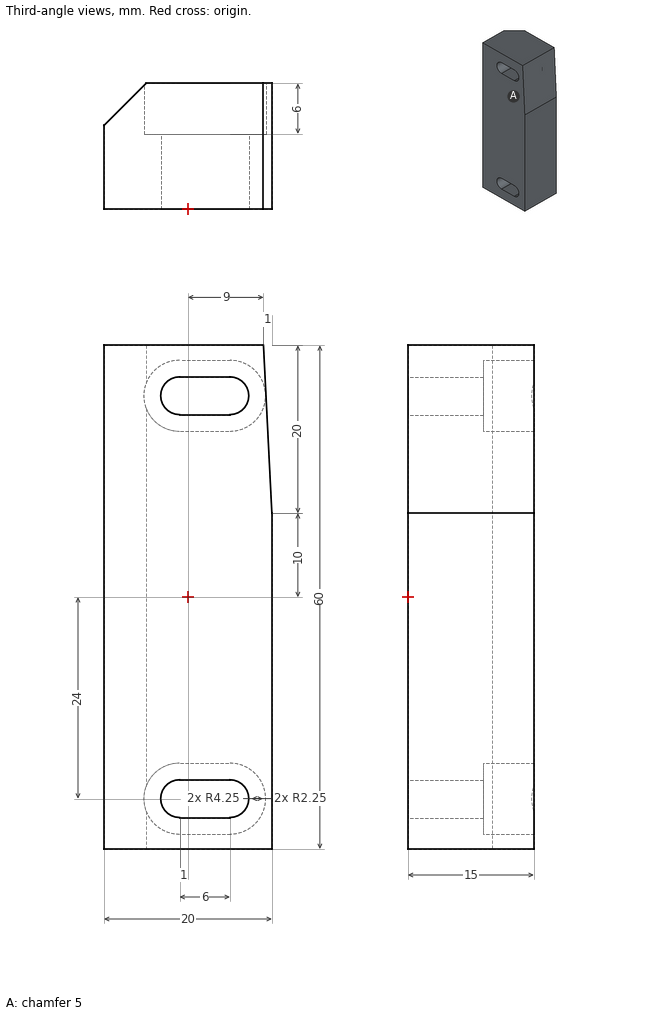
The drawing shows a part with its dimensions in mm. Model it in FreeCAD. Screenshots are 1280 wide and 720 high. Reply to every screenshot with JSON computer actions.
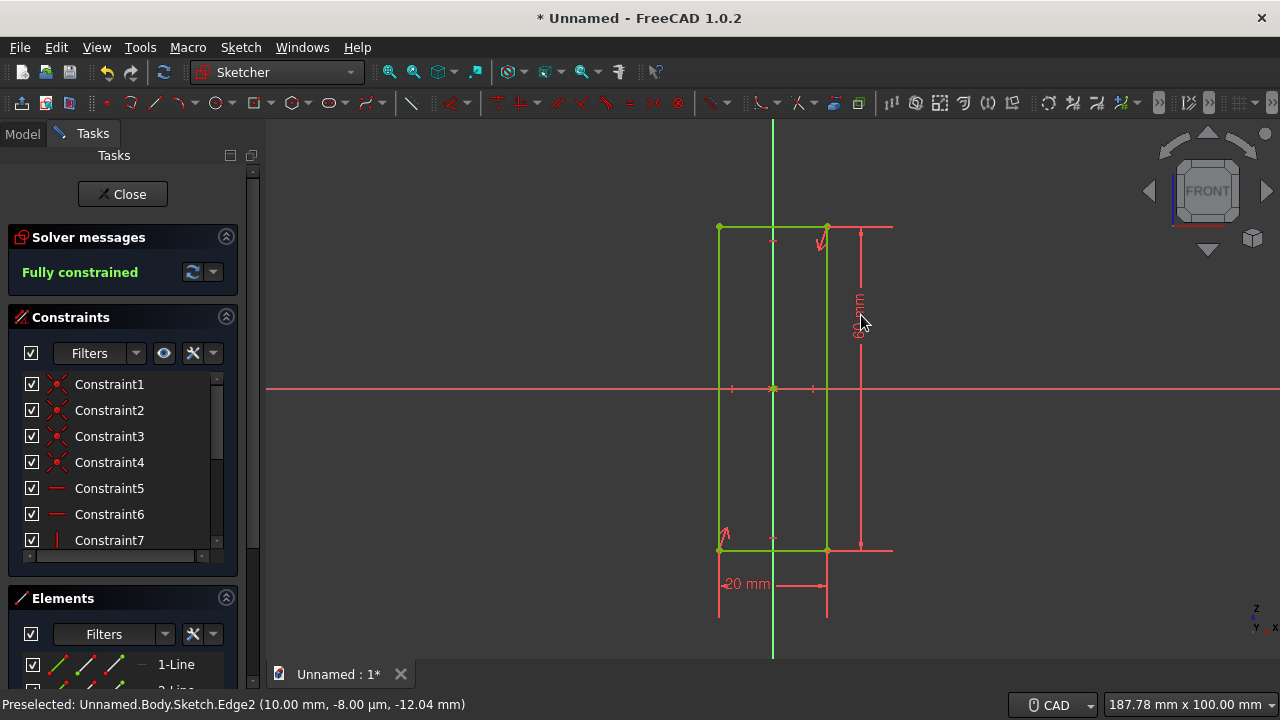
{"action": "left_click", "coordinate": [123, 194]}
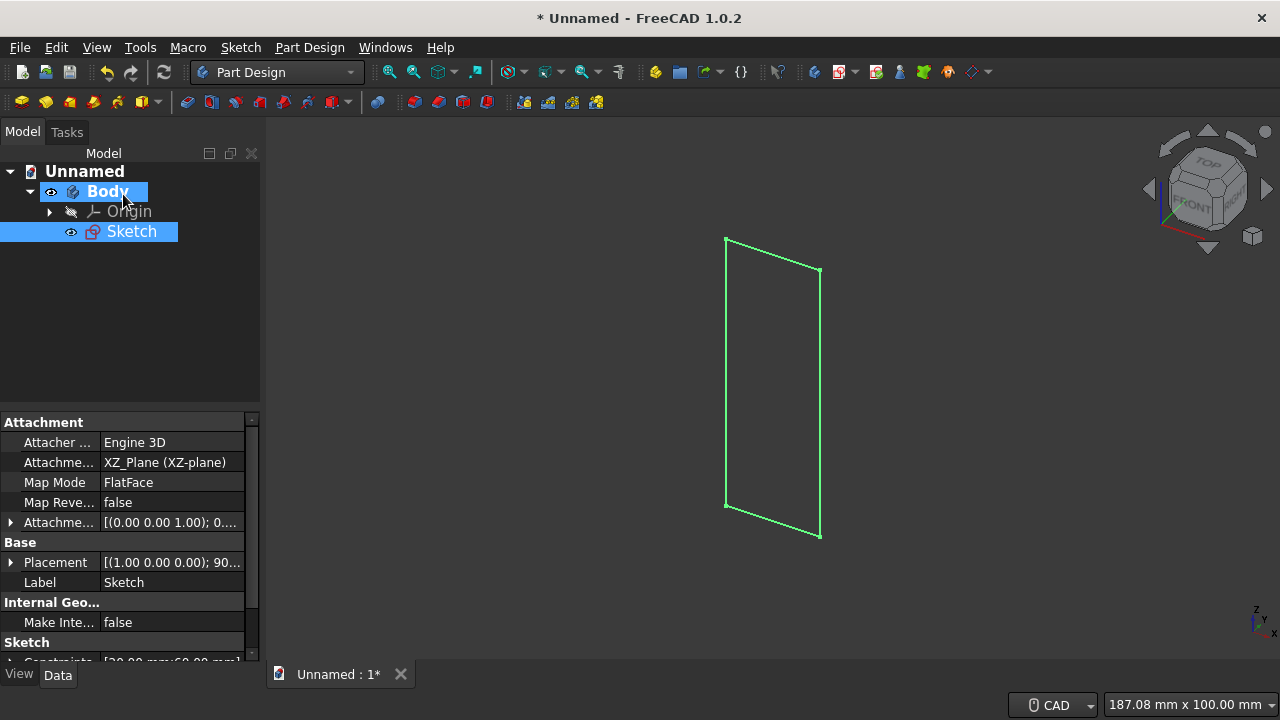
{"action": "left_click", "coordinate": [22, 102]}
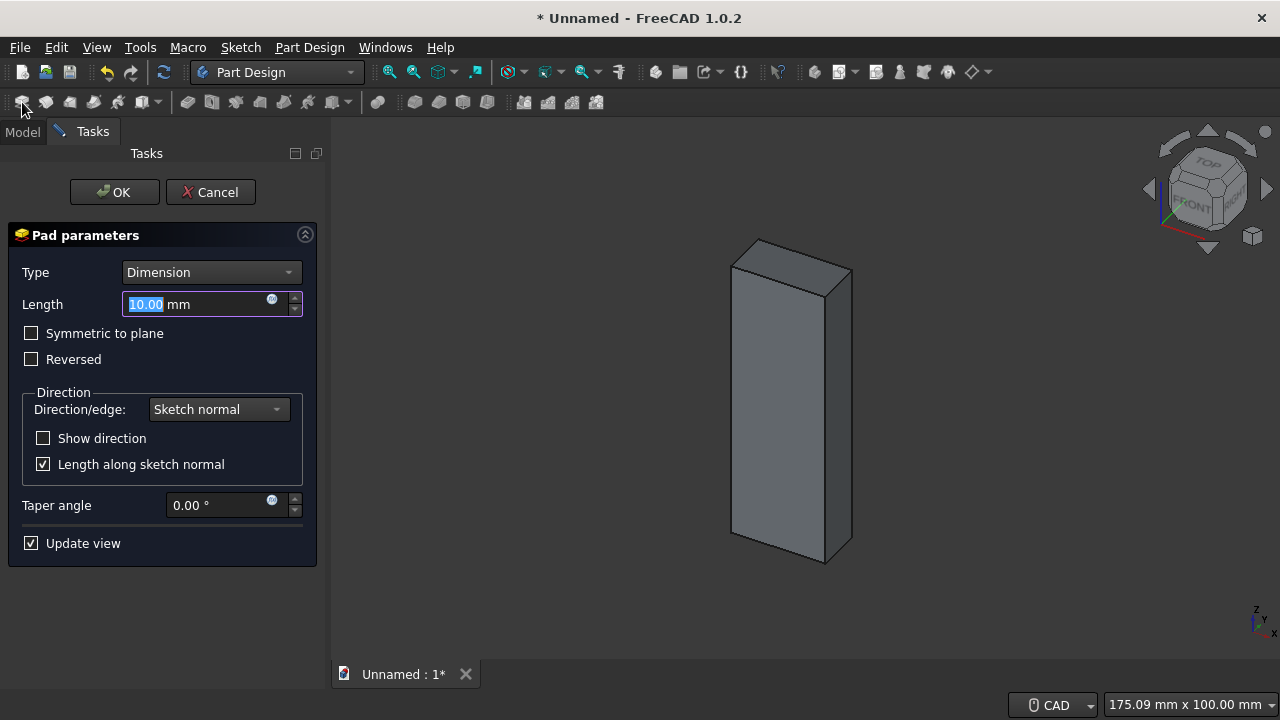
{"action": "type", "text": "15"}
{"action": "key", "text": "Tab"}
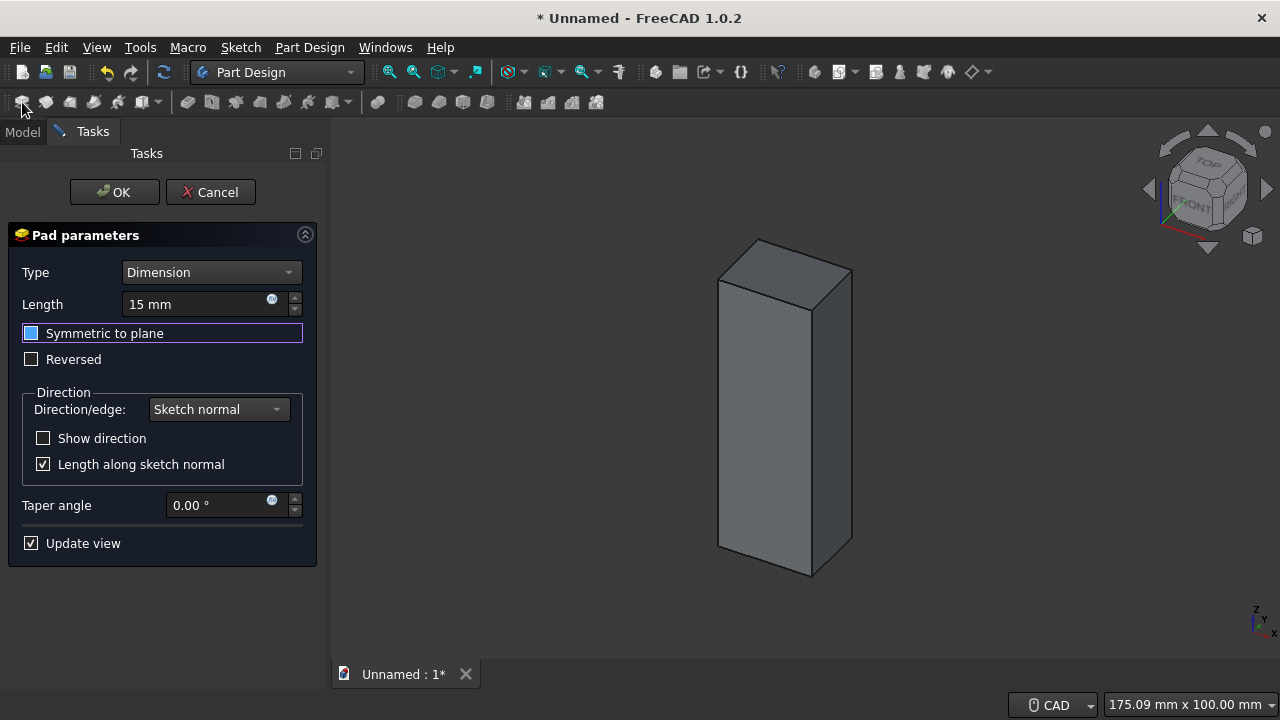
{"action": "left_click", "coordinate": [30, 359]}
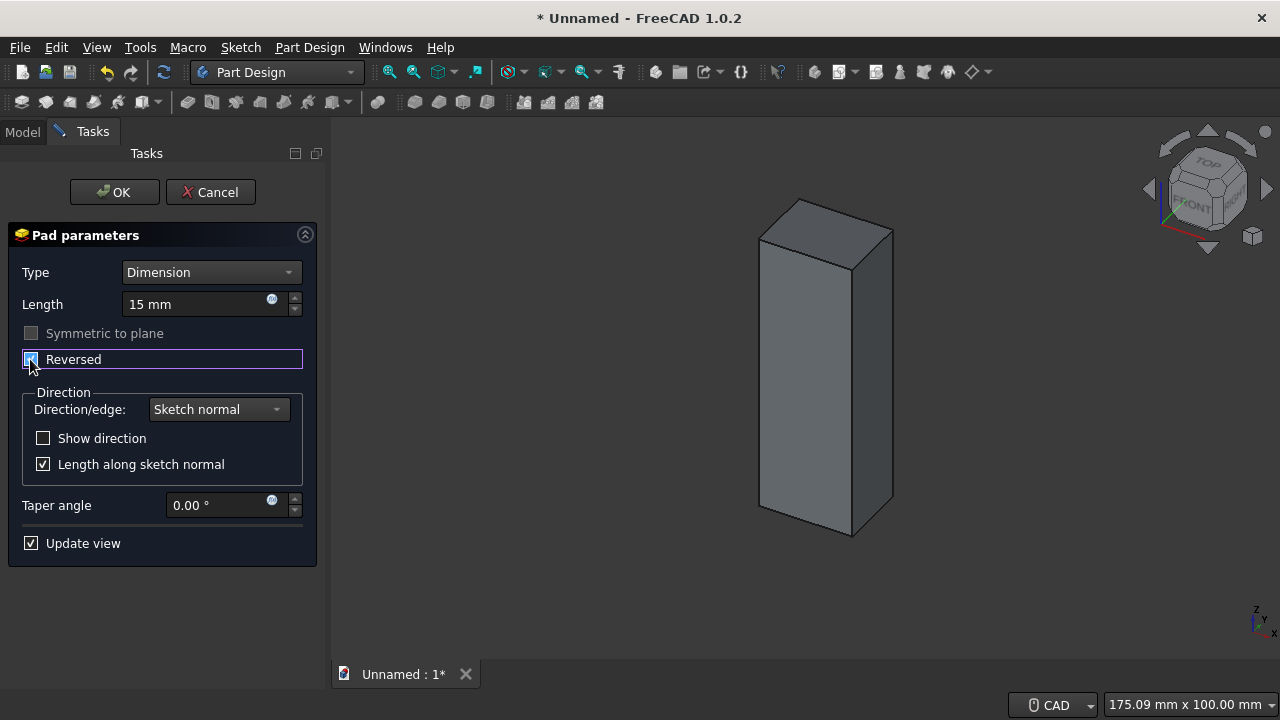
{"action": "left_click", "coordinate": [115, 192]}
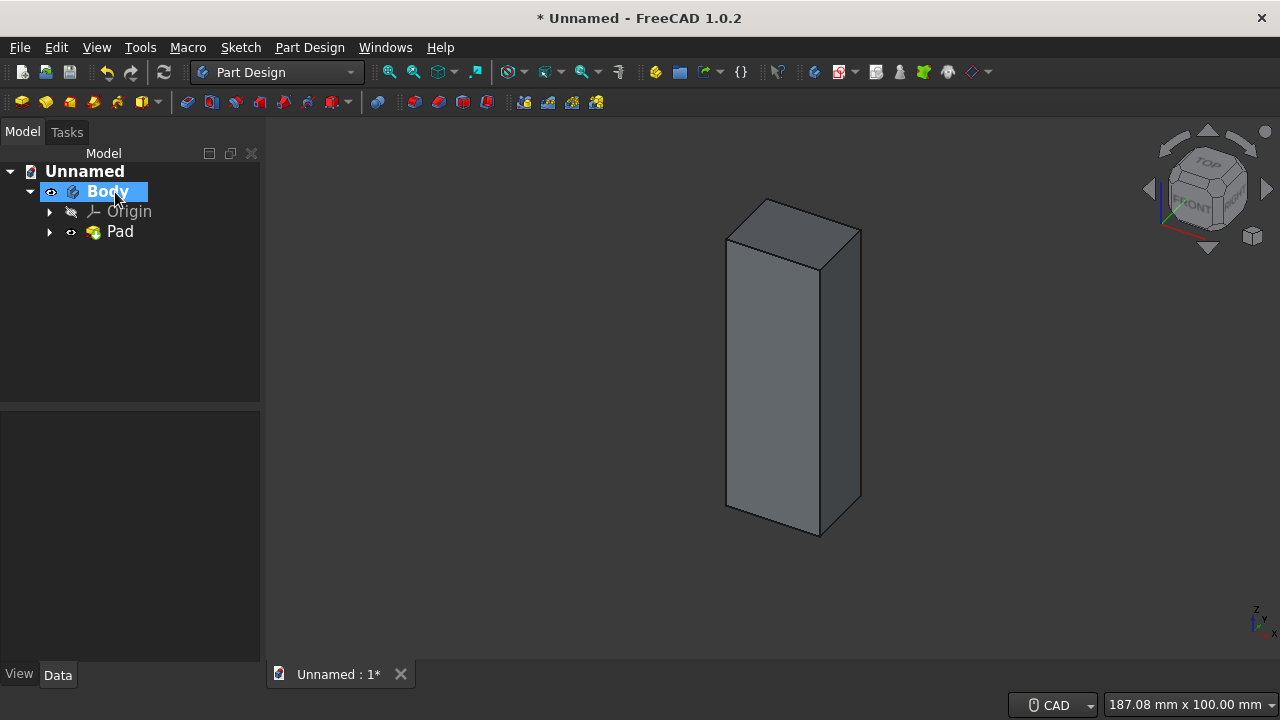
{"action": "key", "text": "0"}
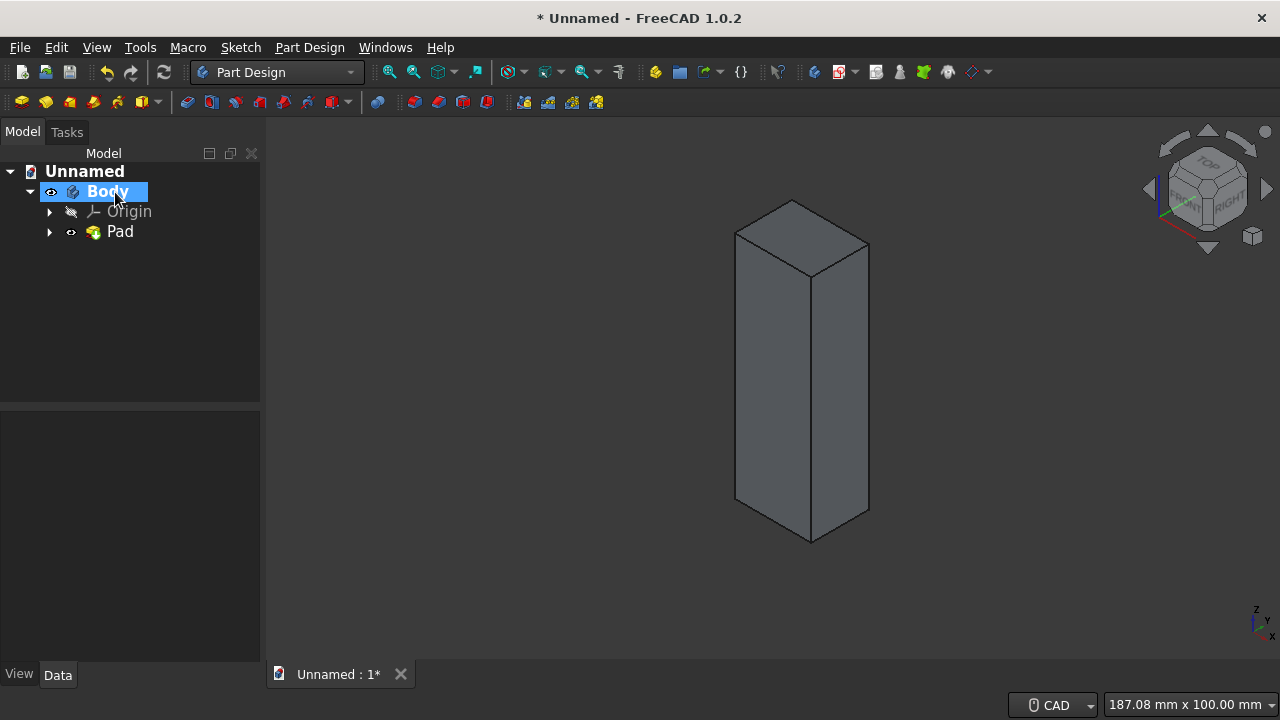
{"action": "key", "text": "2"}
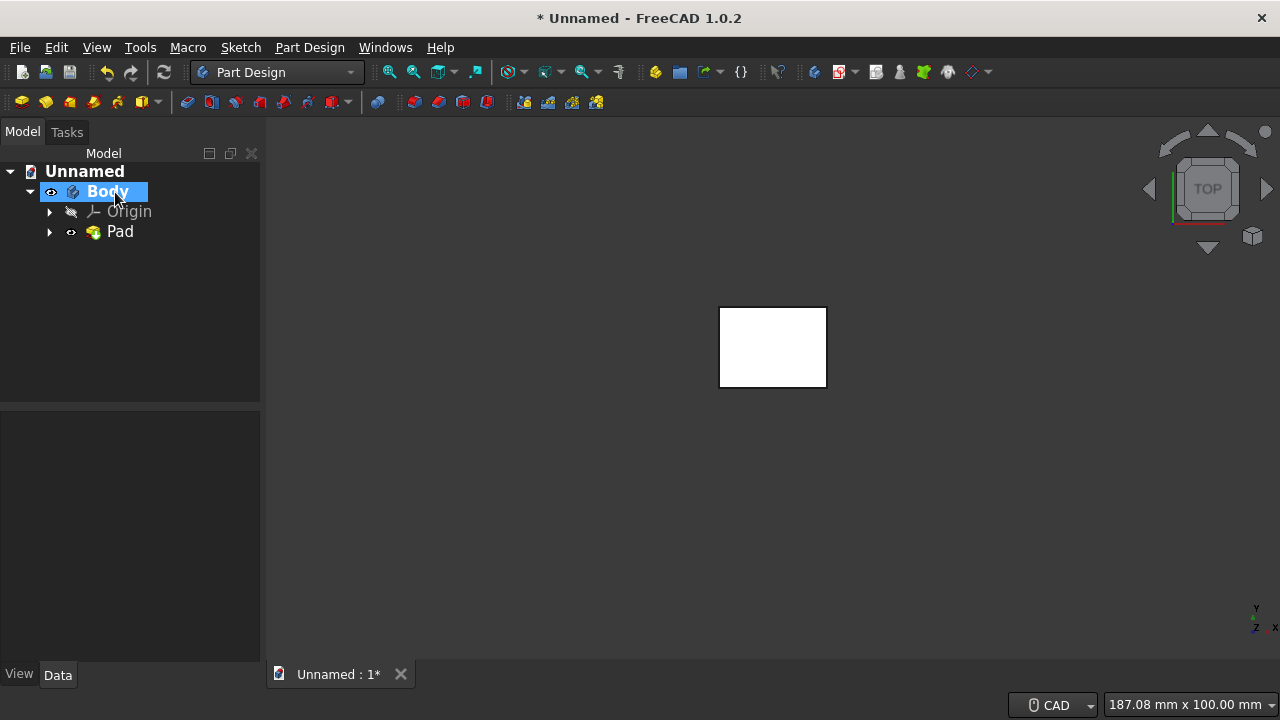
{"action": "left_click", "coordinate": [390, 72]}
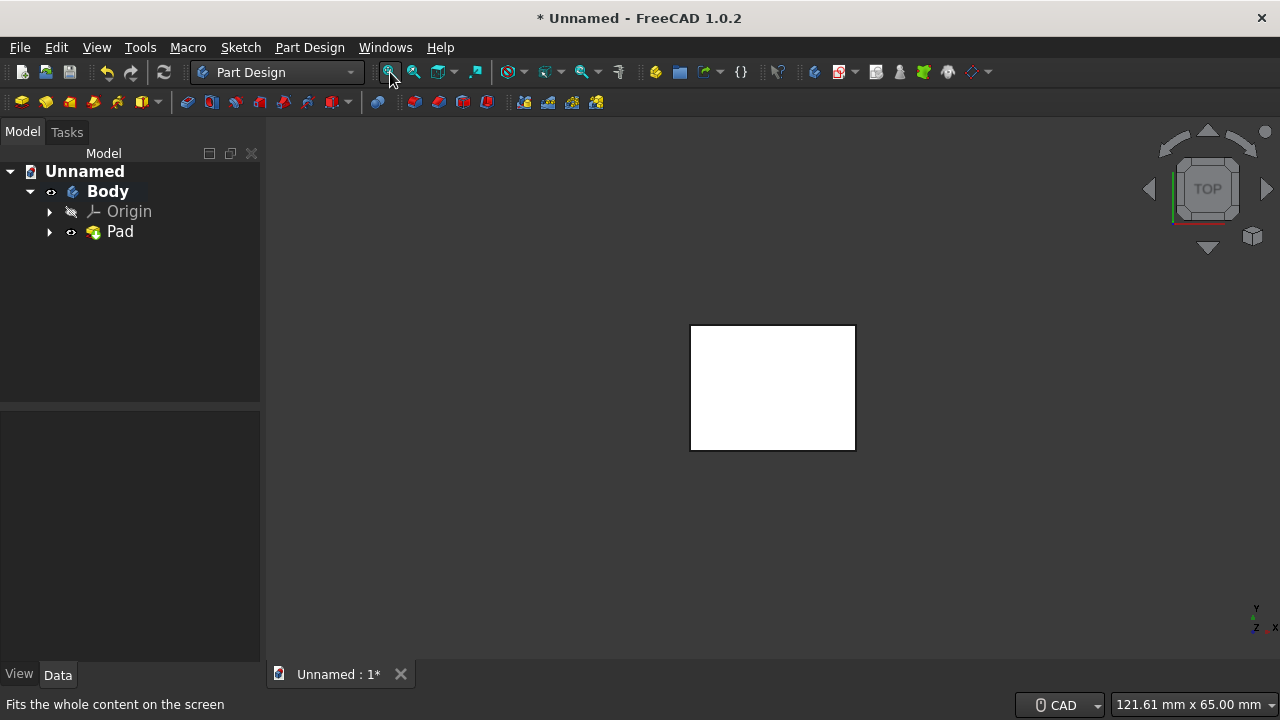
{"action": "key", "text": "1"}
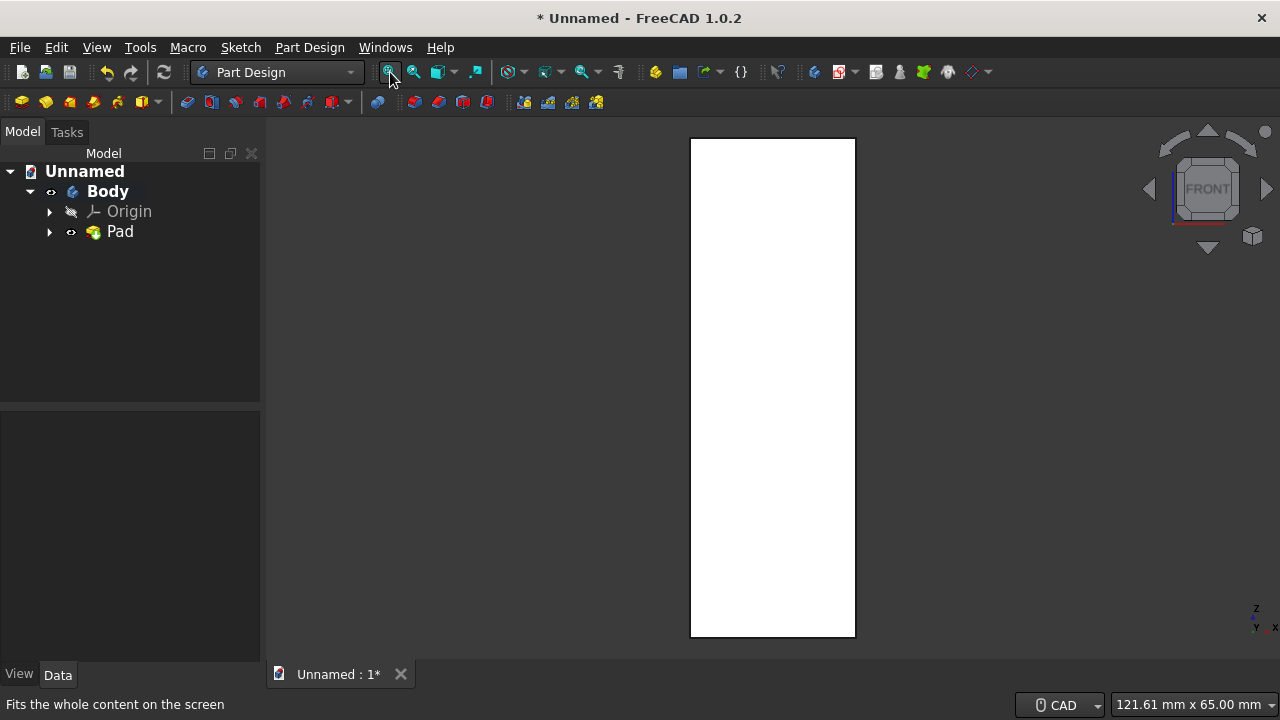
{"action": "key", "text": "3"}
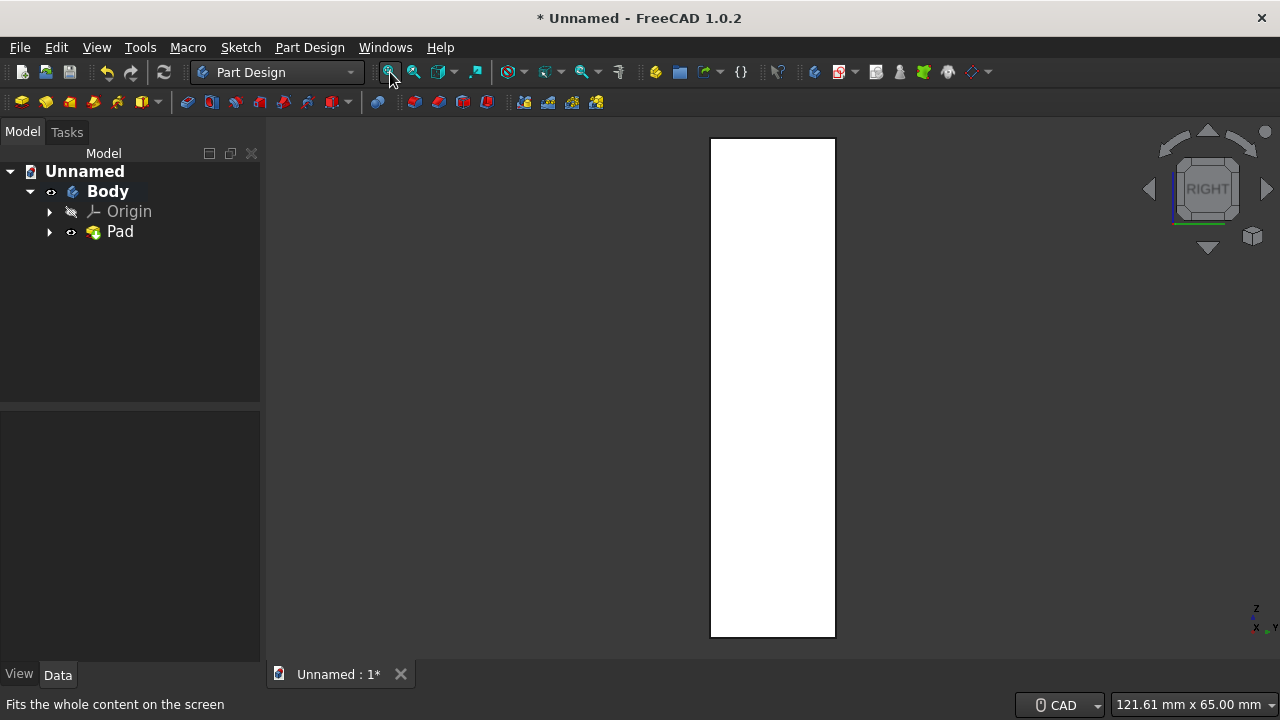
{"action": "key", "text": "5"}